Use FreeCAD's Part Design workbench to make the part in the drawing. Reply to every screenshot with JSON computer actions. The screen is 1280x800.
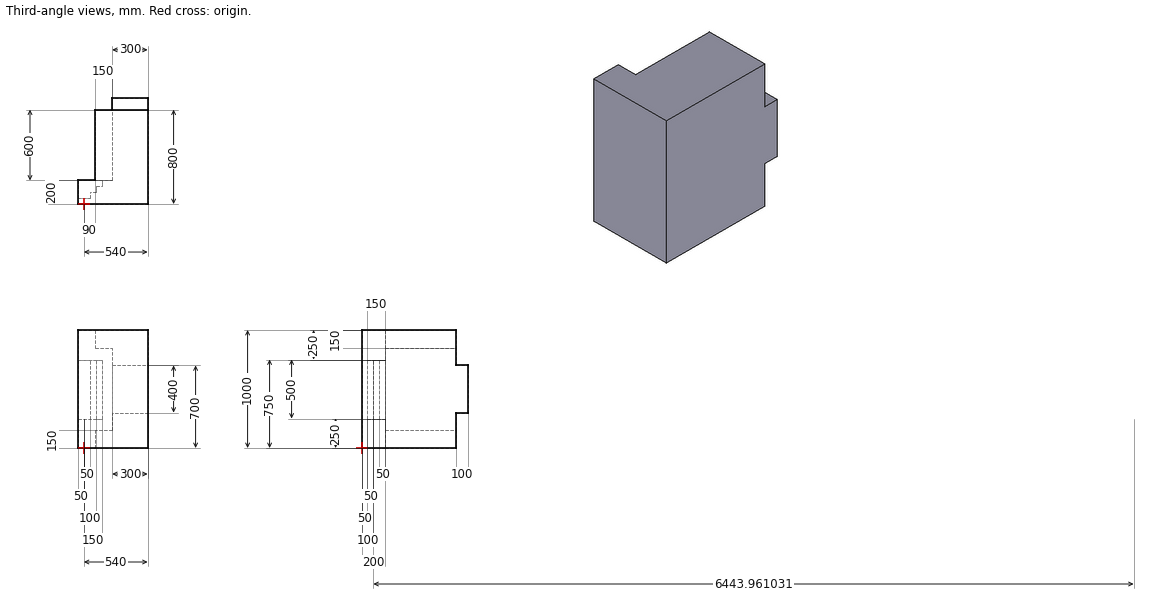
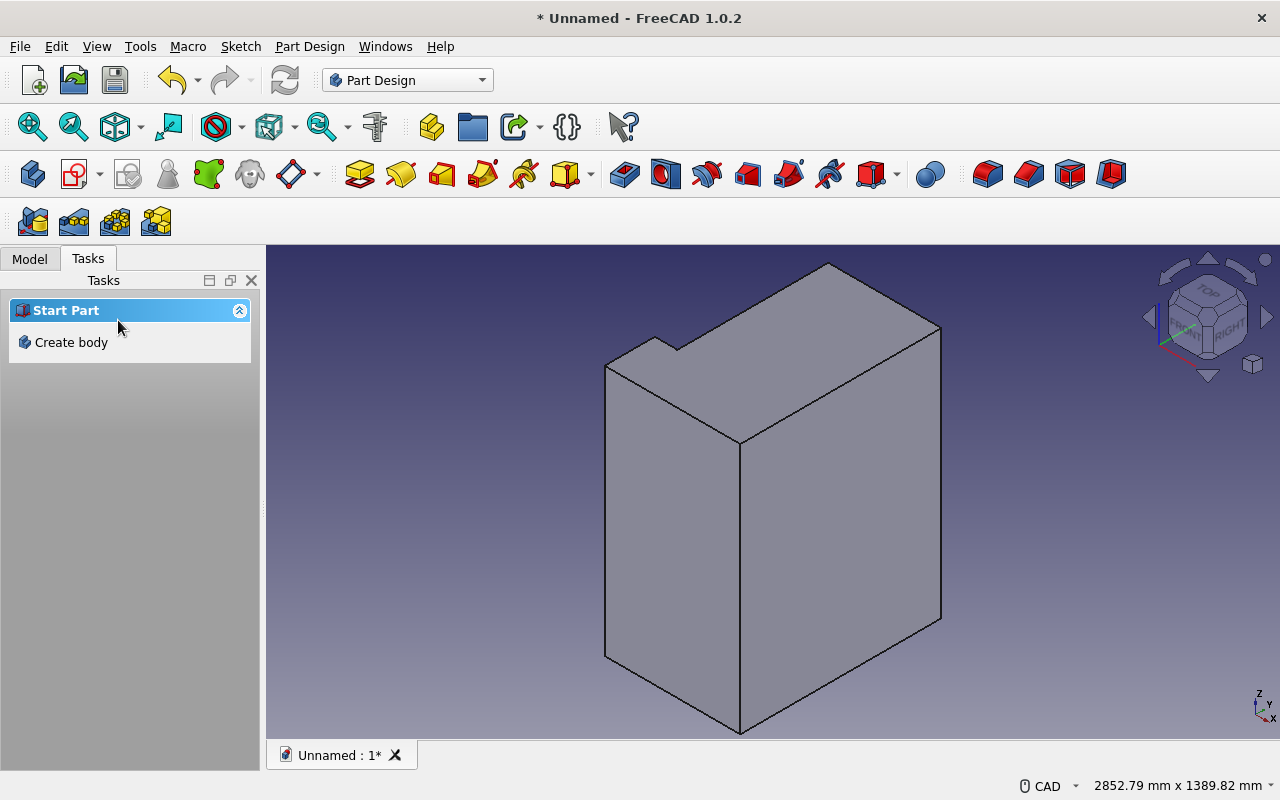
{"action": "key", "text": "4"}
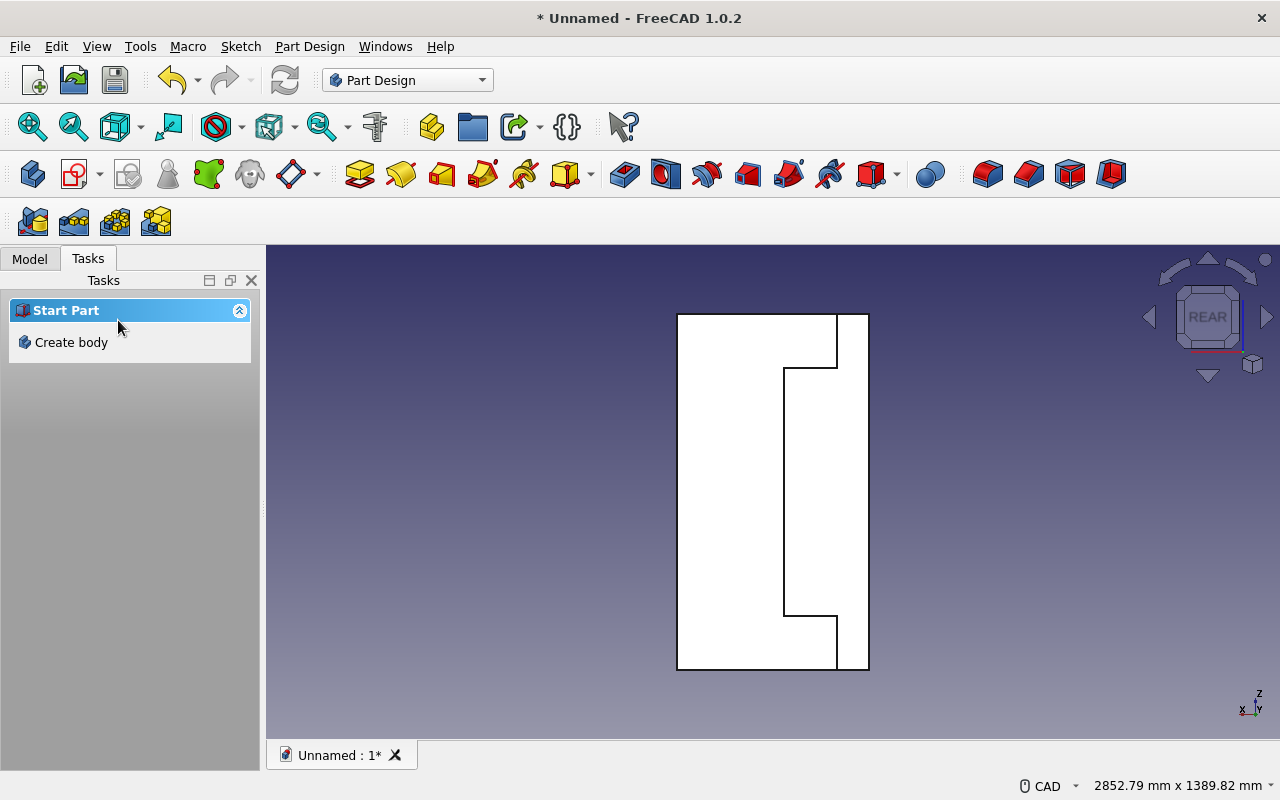
{"action": "left_click", "coordinate": [734, 389]}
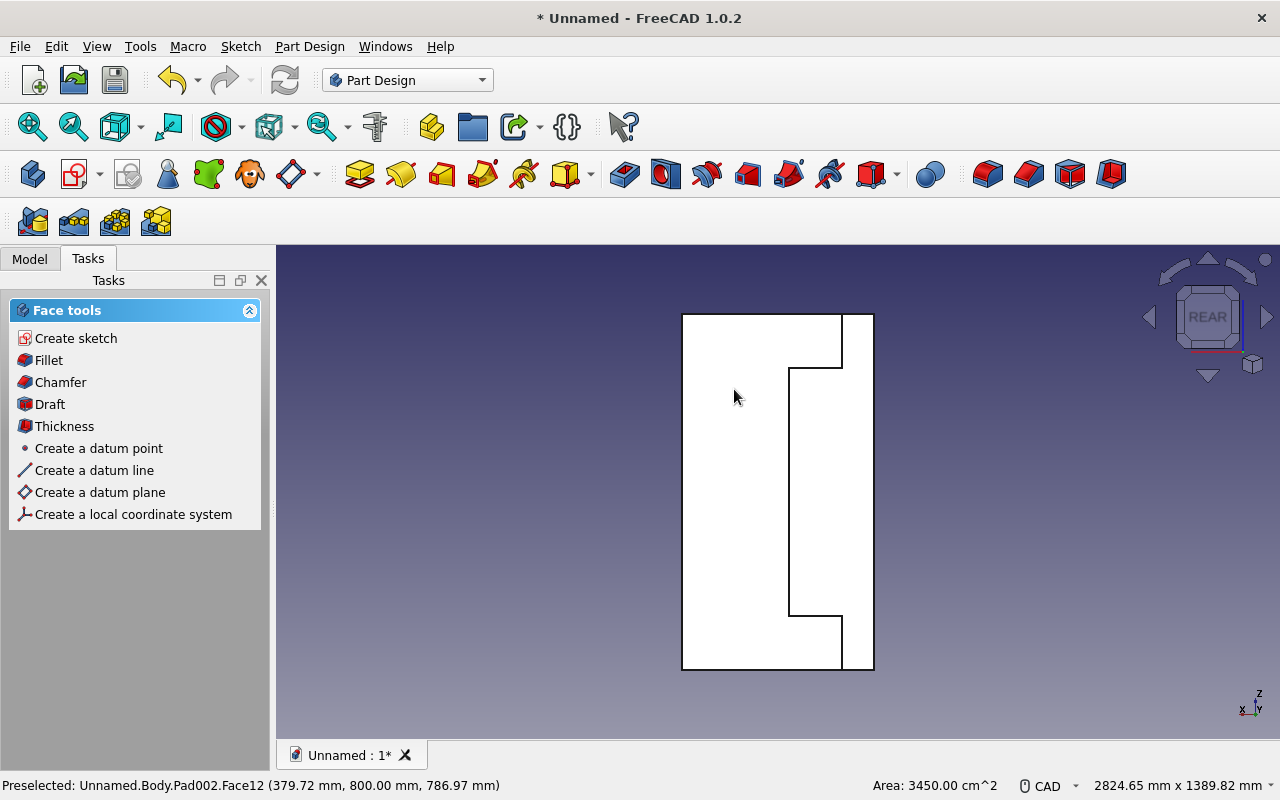
{"action": "left_click", "coordinate": [74, 174]}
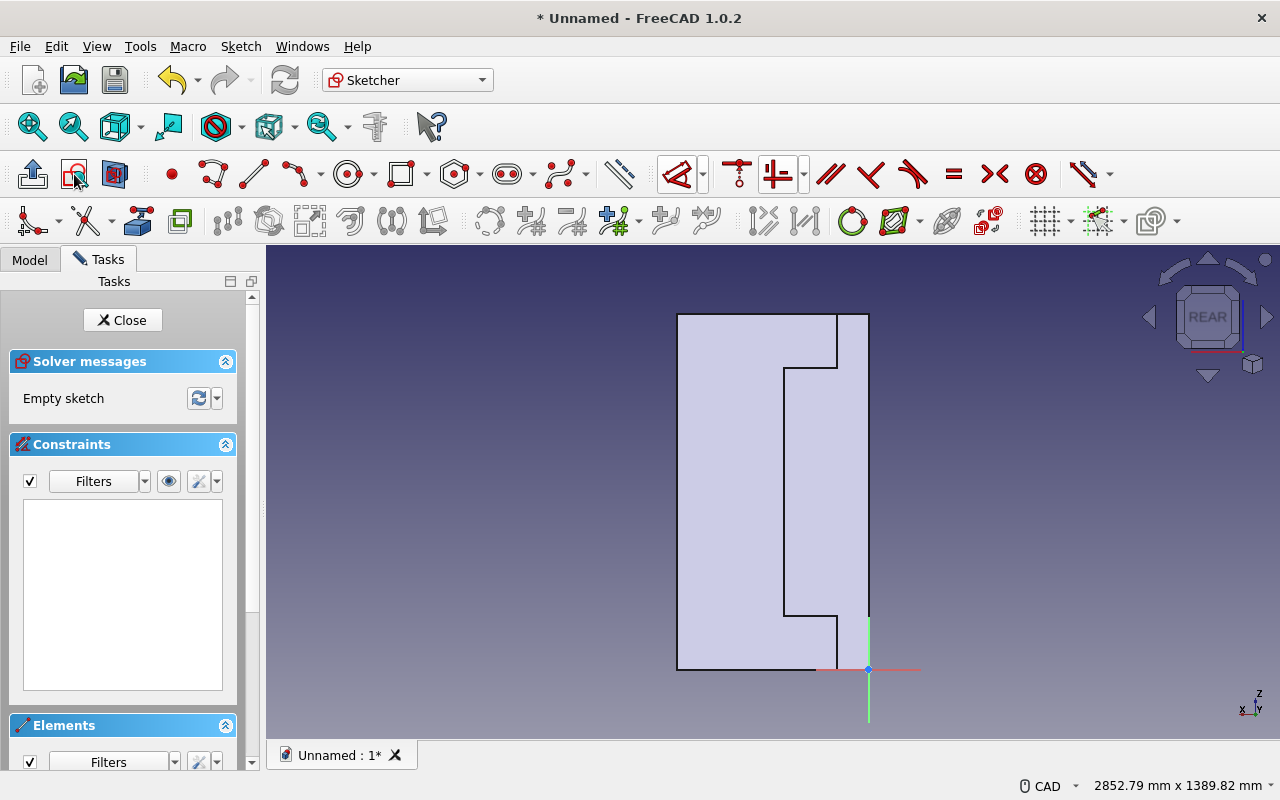
{"action": "left_click", "coordinate": [400, 174]}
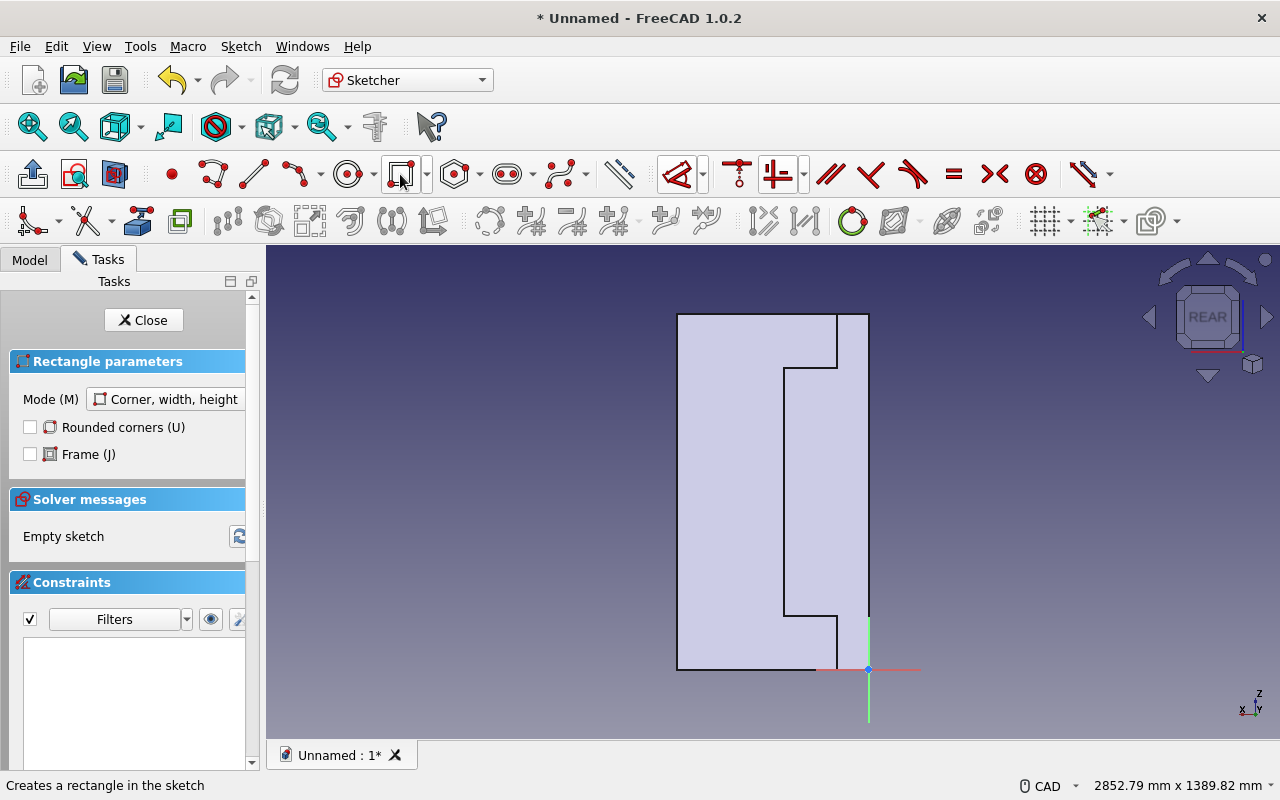
{"action": "left_click", "coordinate": [677, 421]}
{"action": "left_click", "coordinate": [784, 563]}
{"action": "key", "text": "Escape"}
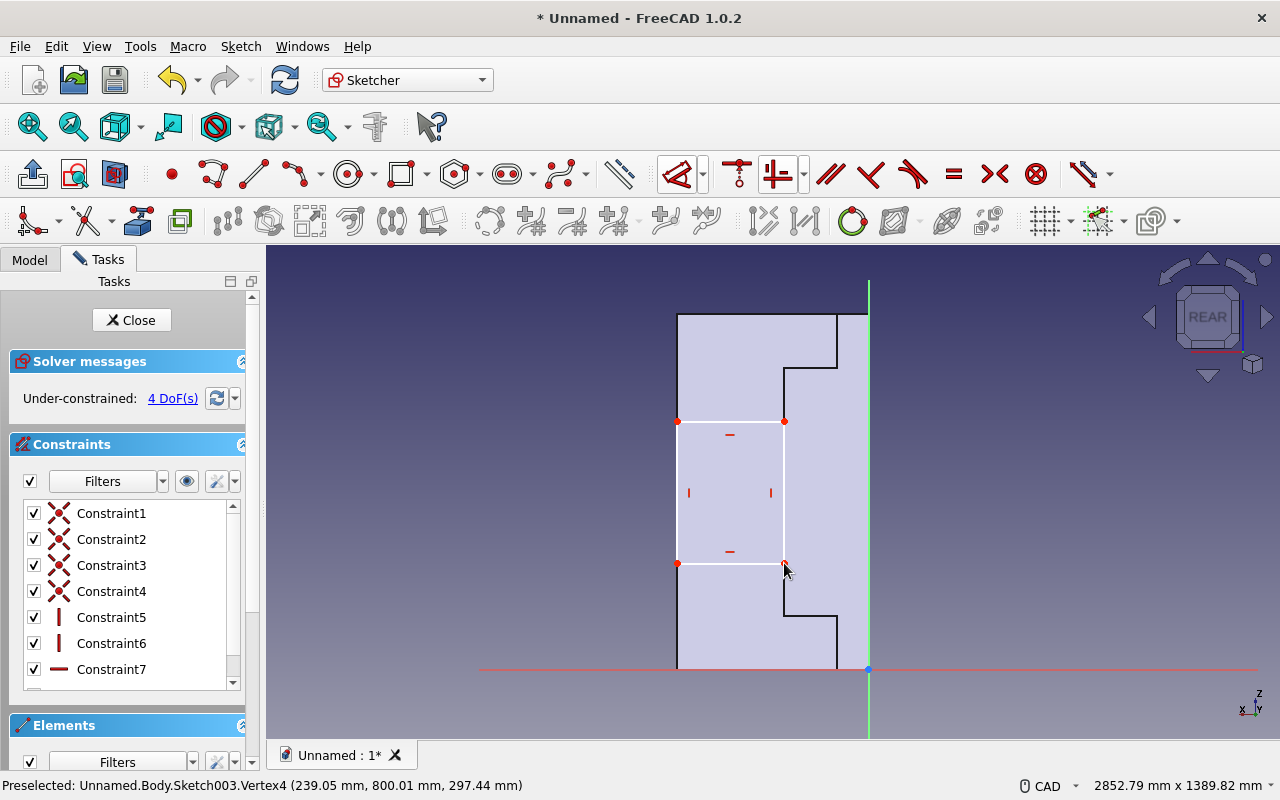
{"action": "left_click", "coordinate": [677, 465]}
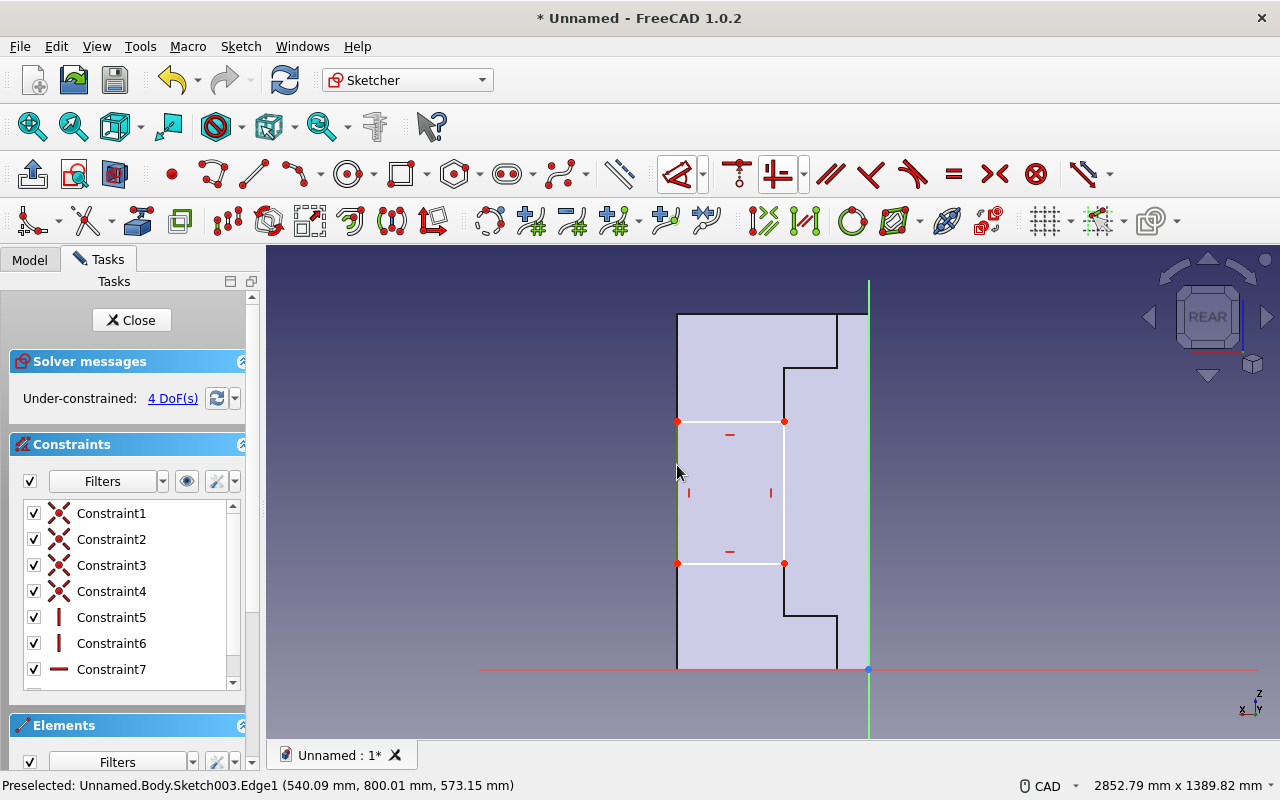
{"action": "key", "text": "i"}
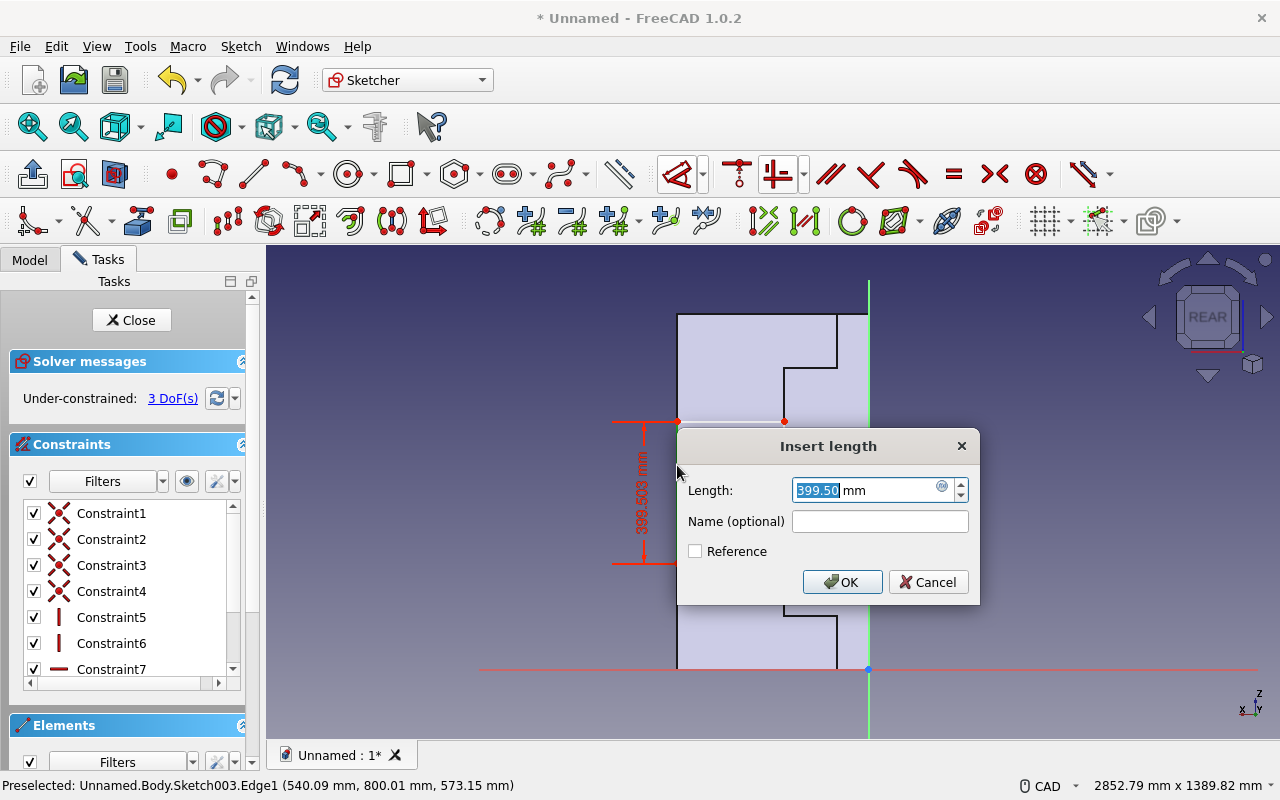
{"action": "type", "text": "400"}
{"action": "key", "text": "Return"}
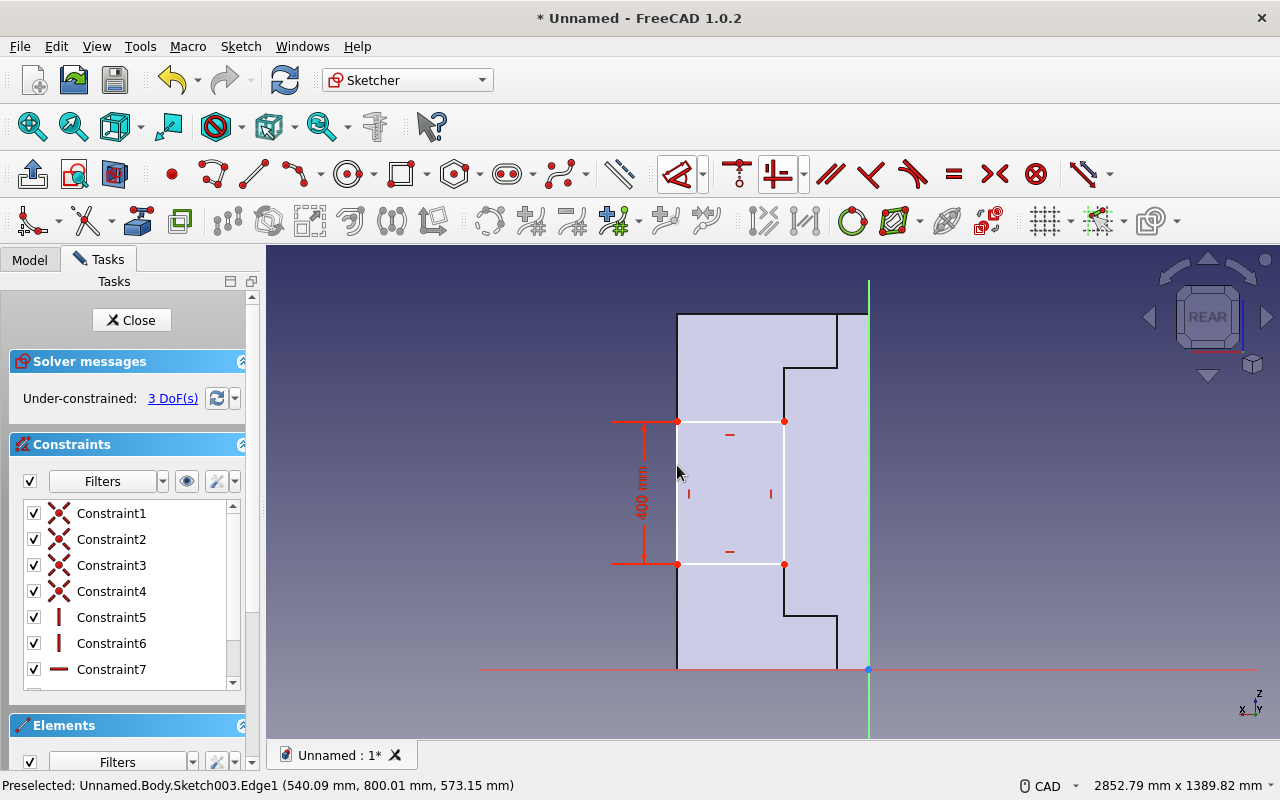
{"action": "left_click", "coordinate": [709, 564]}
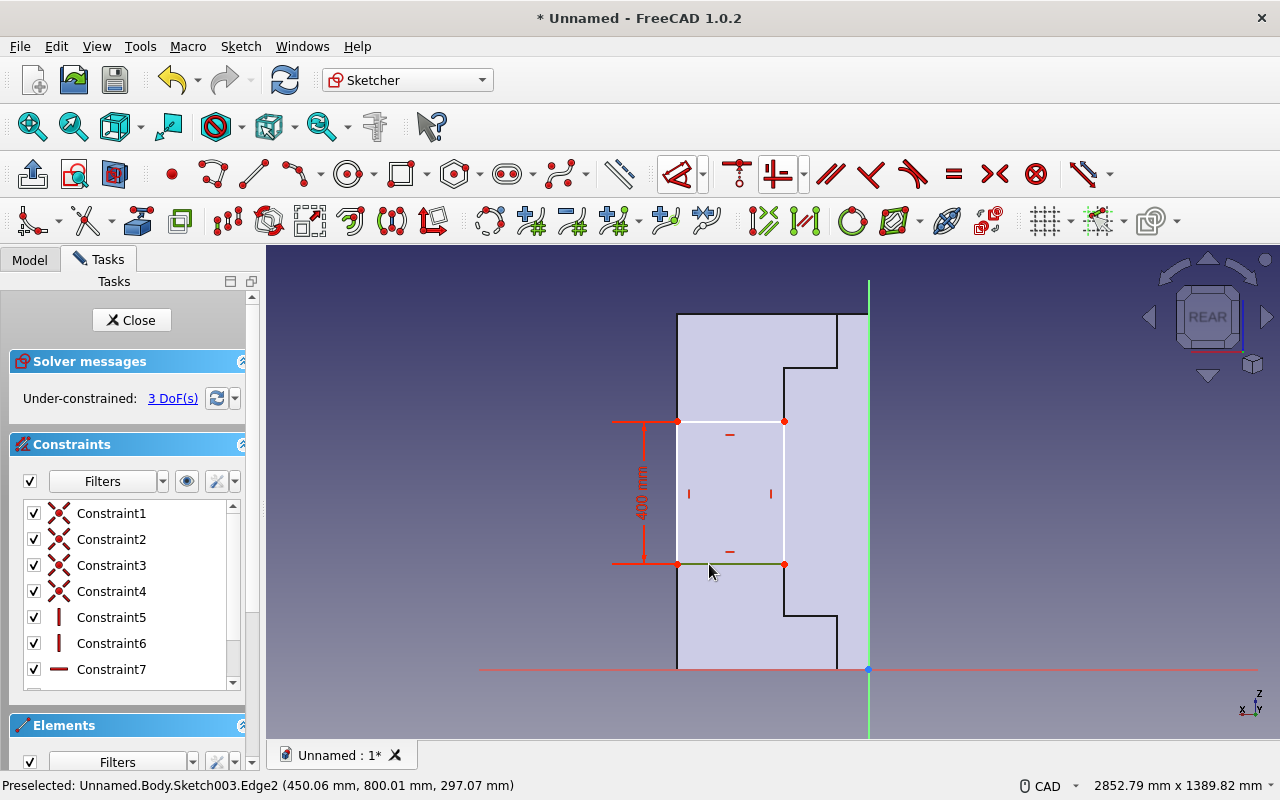
{"action": "key", "text": "l"}